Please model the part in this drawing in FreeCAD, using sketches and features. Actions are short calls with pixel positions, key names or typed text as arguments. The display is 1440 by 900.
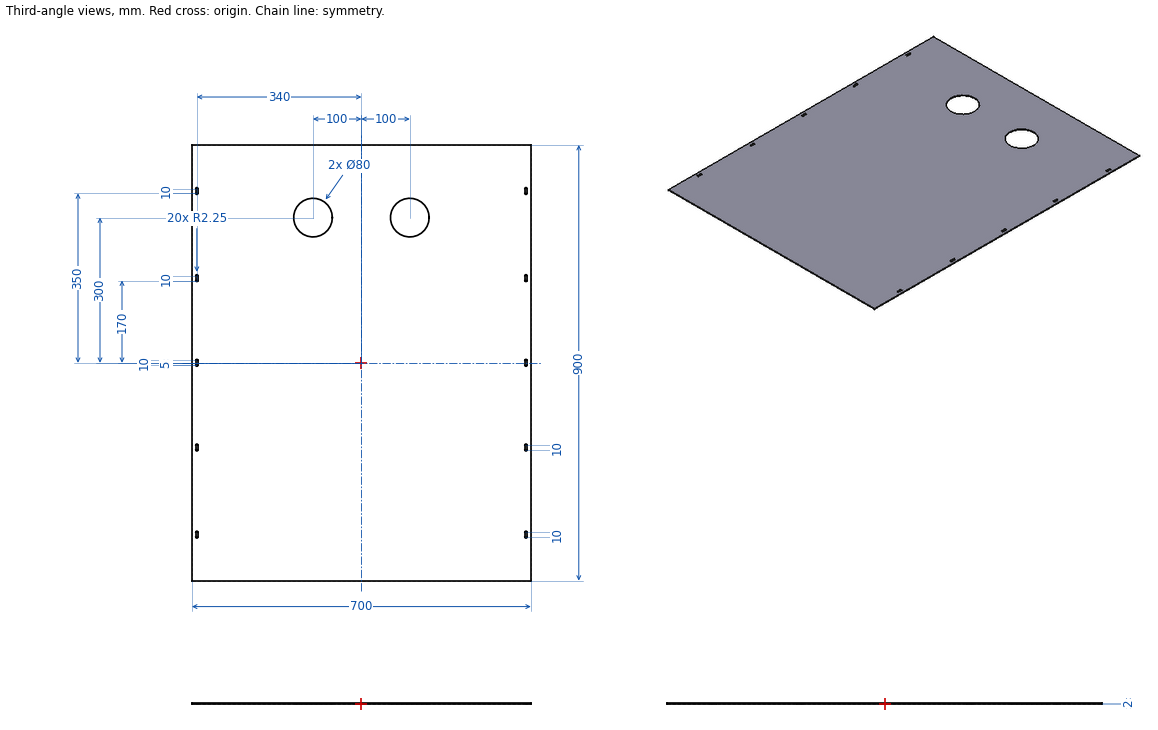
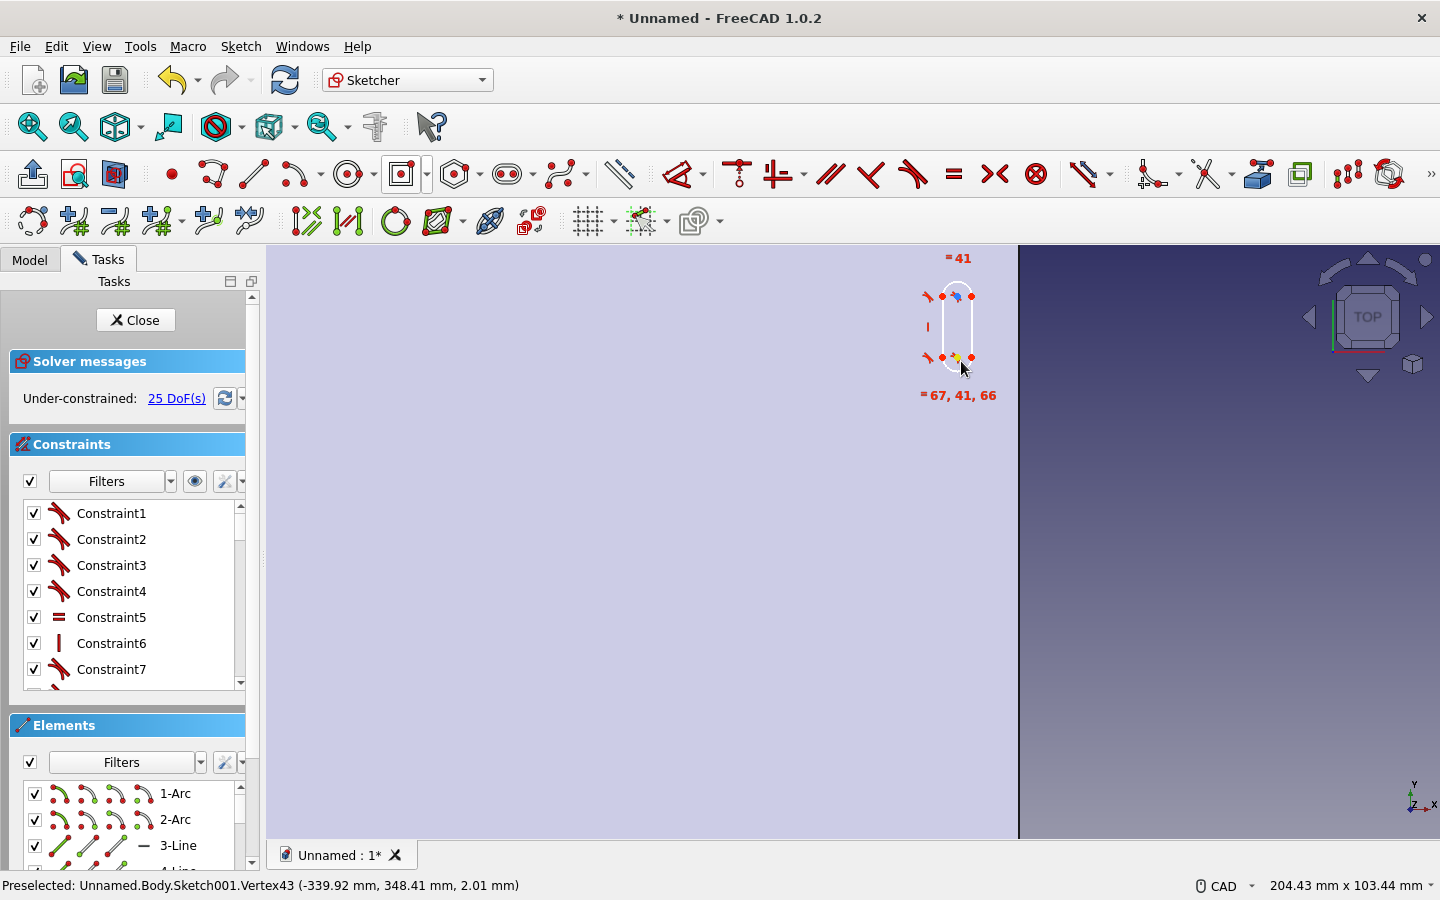
click(957, 357)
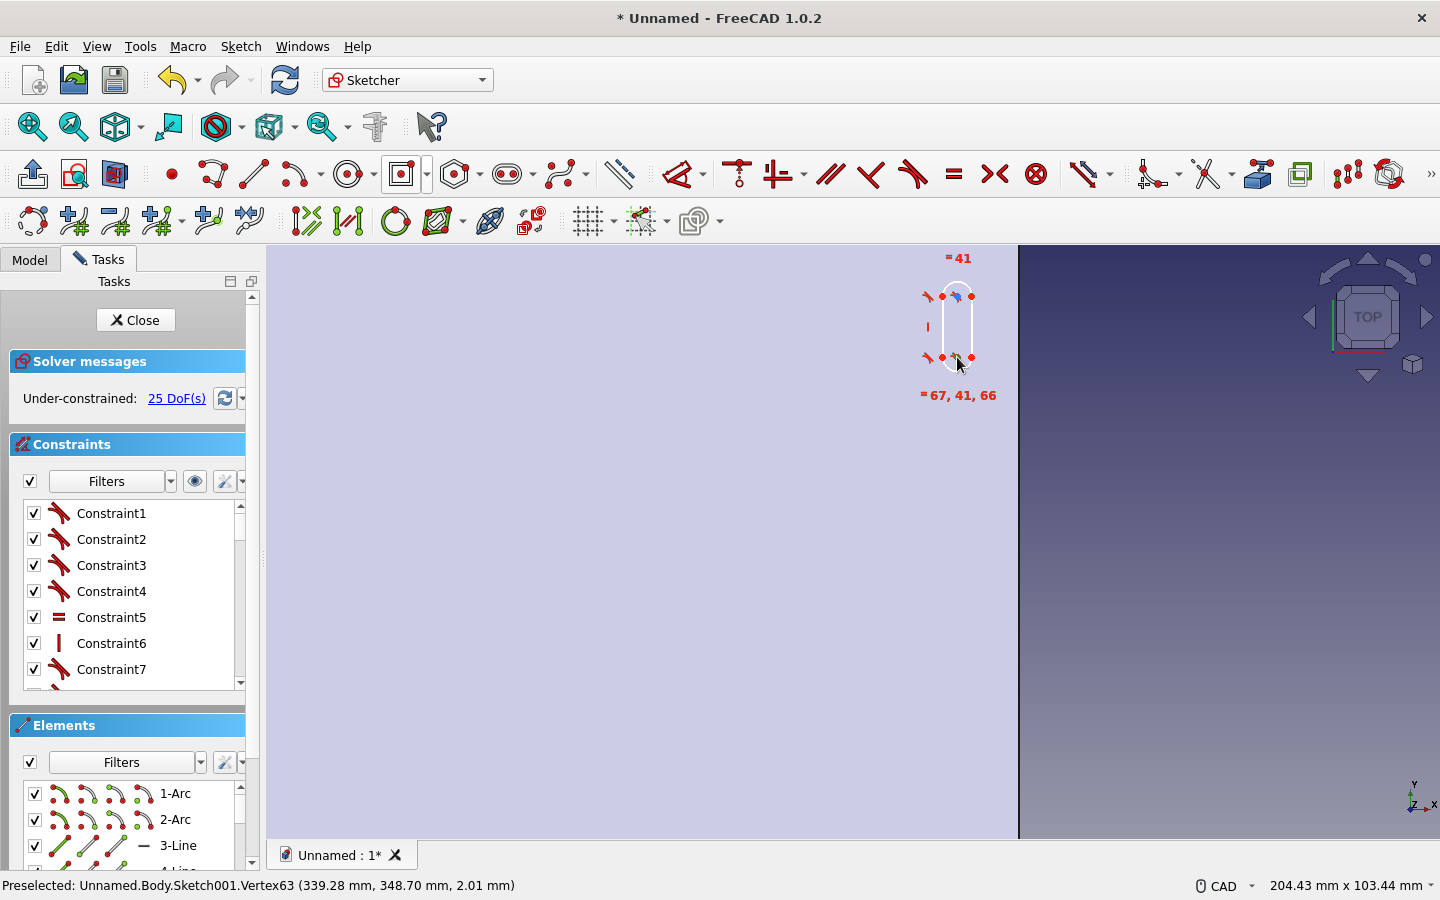
scroll(962, 361, down, 12)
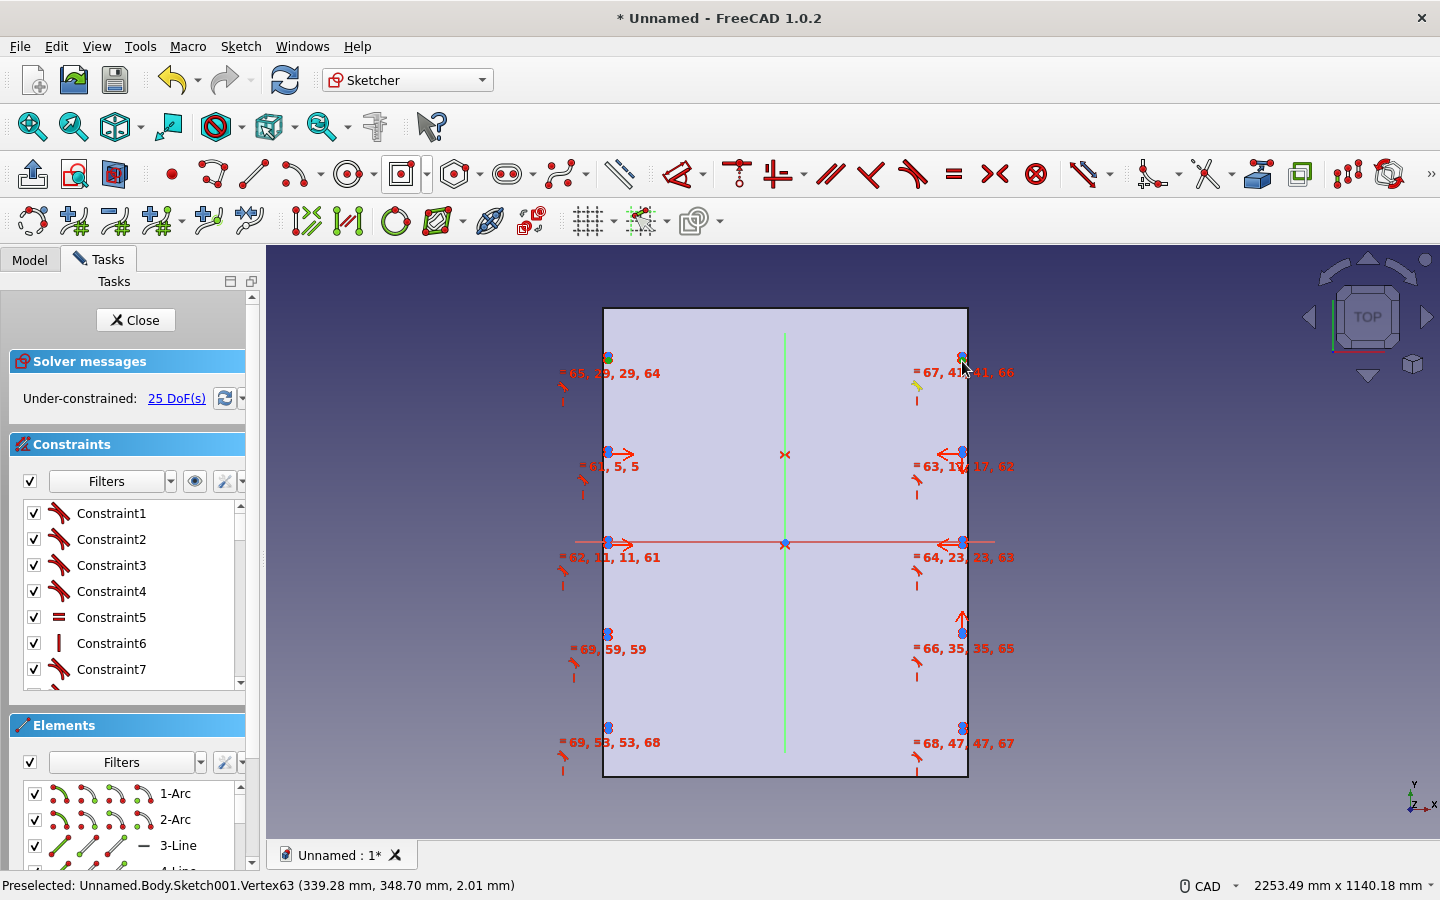
click(785, 734)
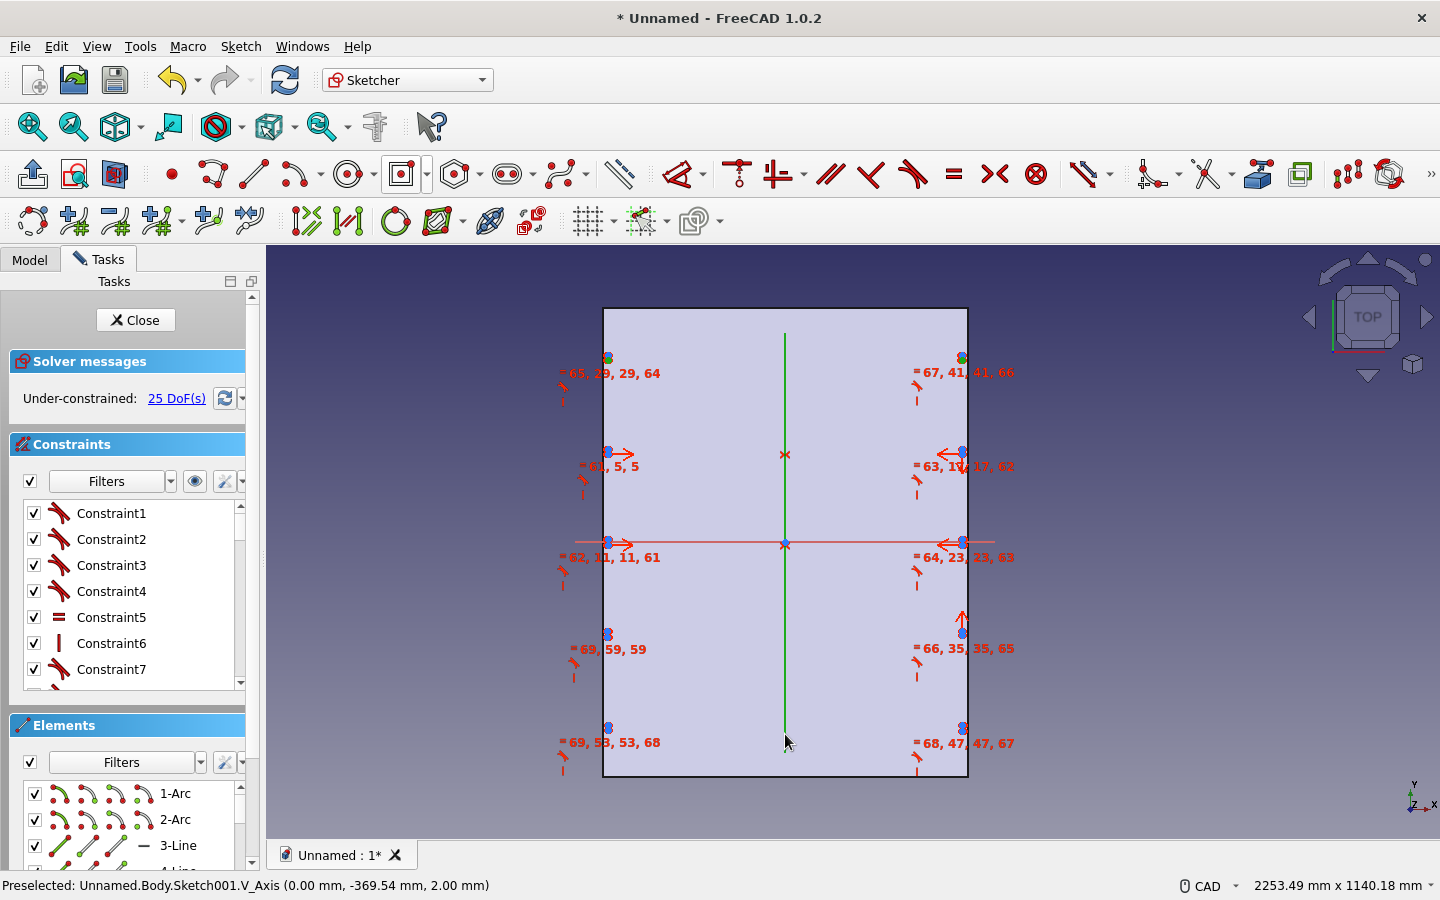
key(s)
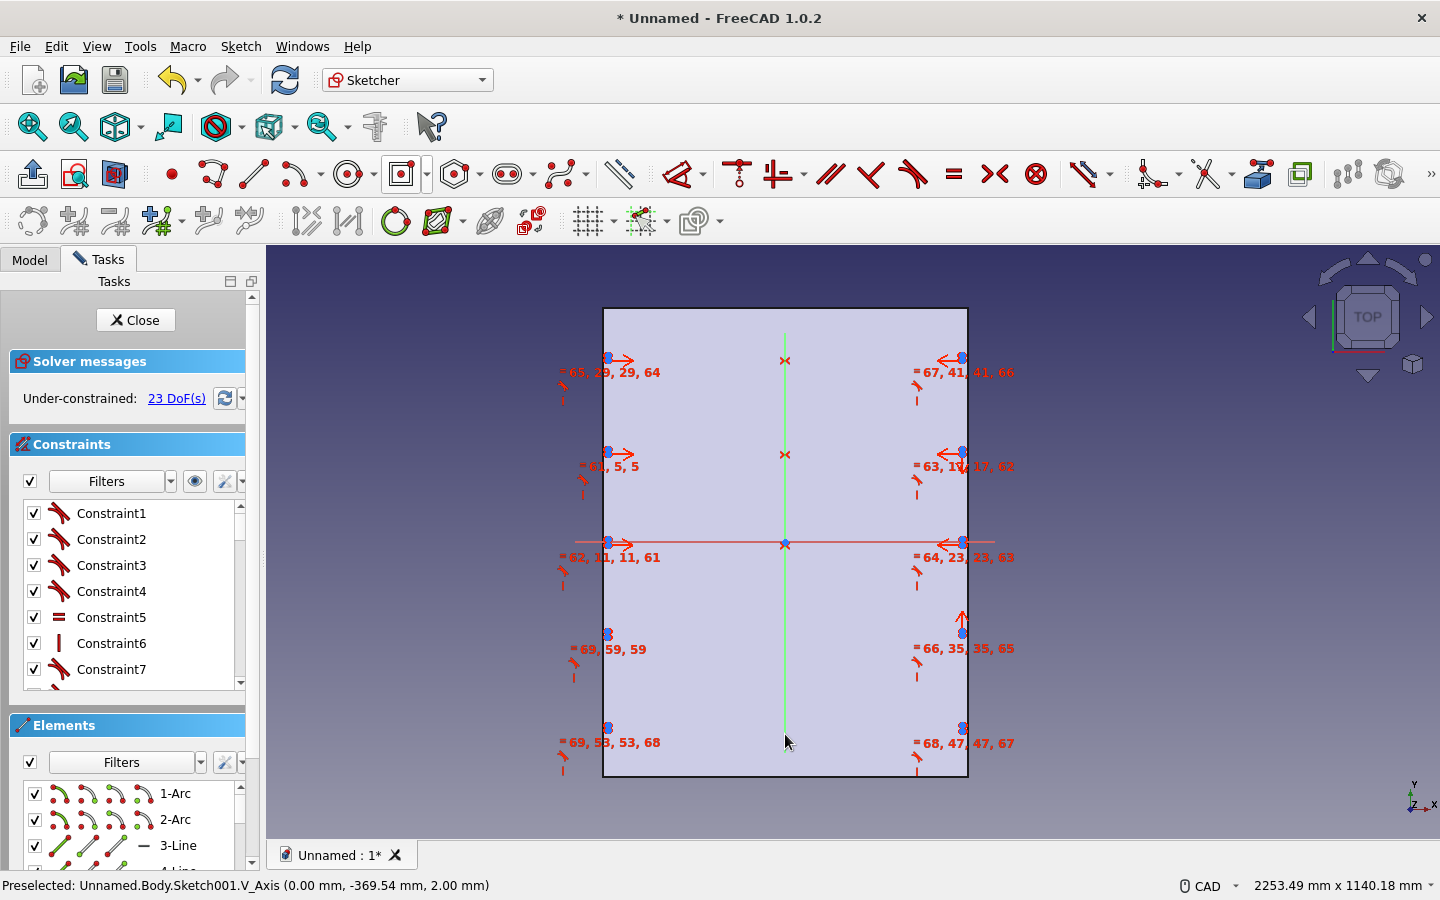
scroll(962, 355, up, 11)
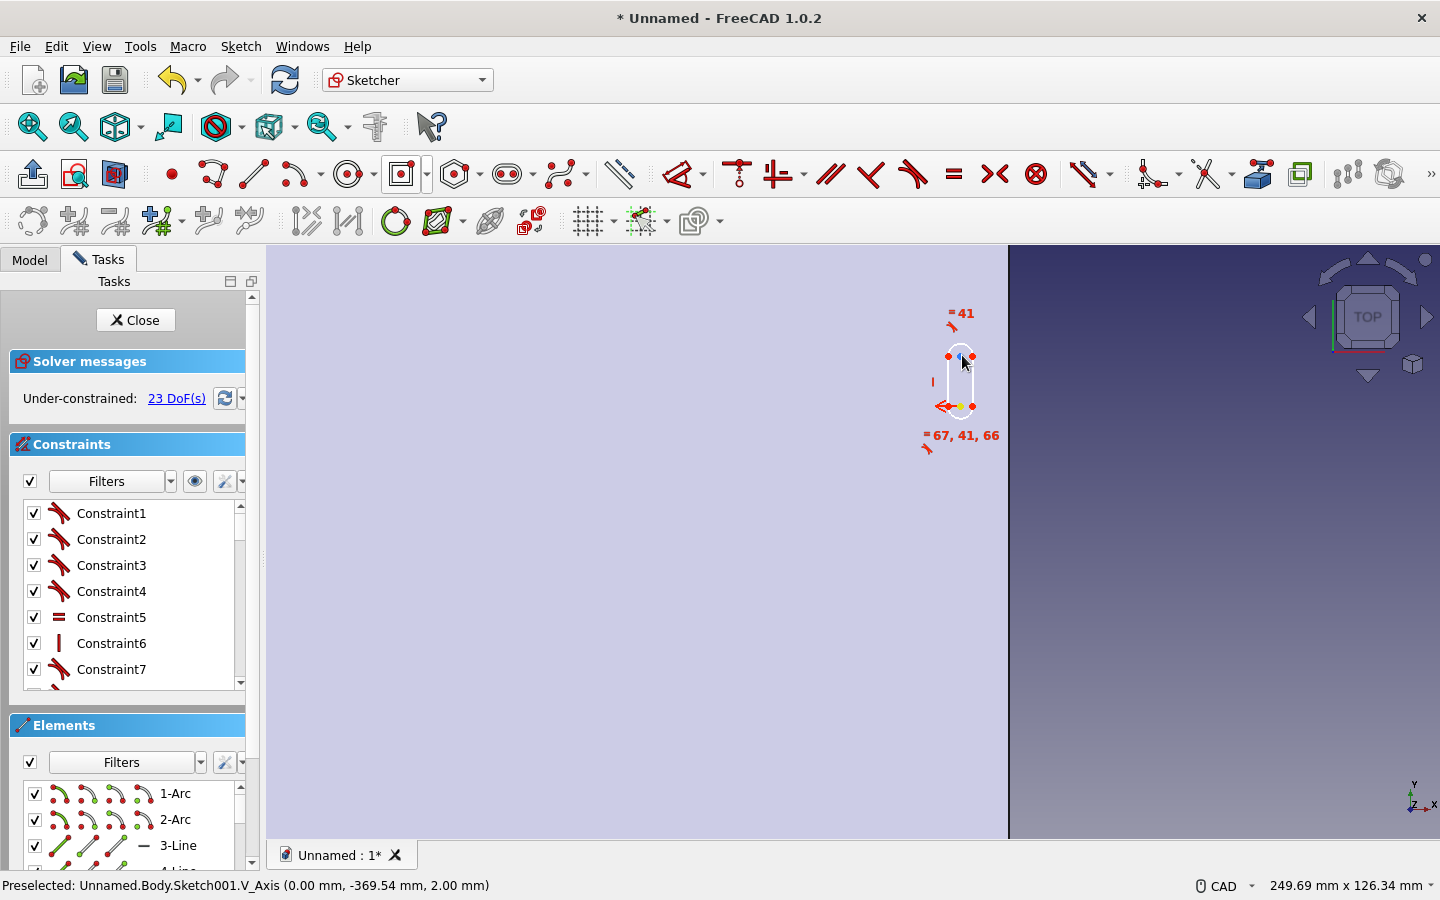
click(961, 356)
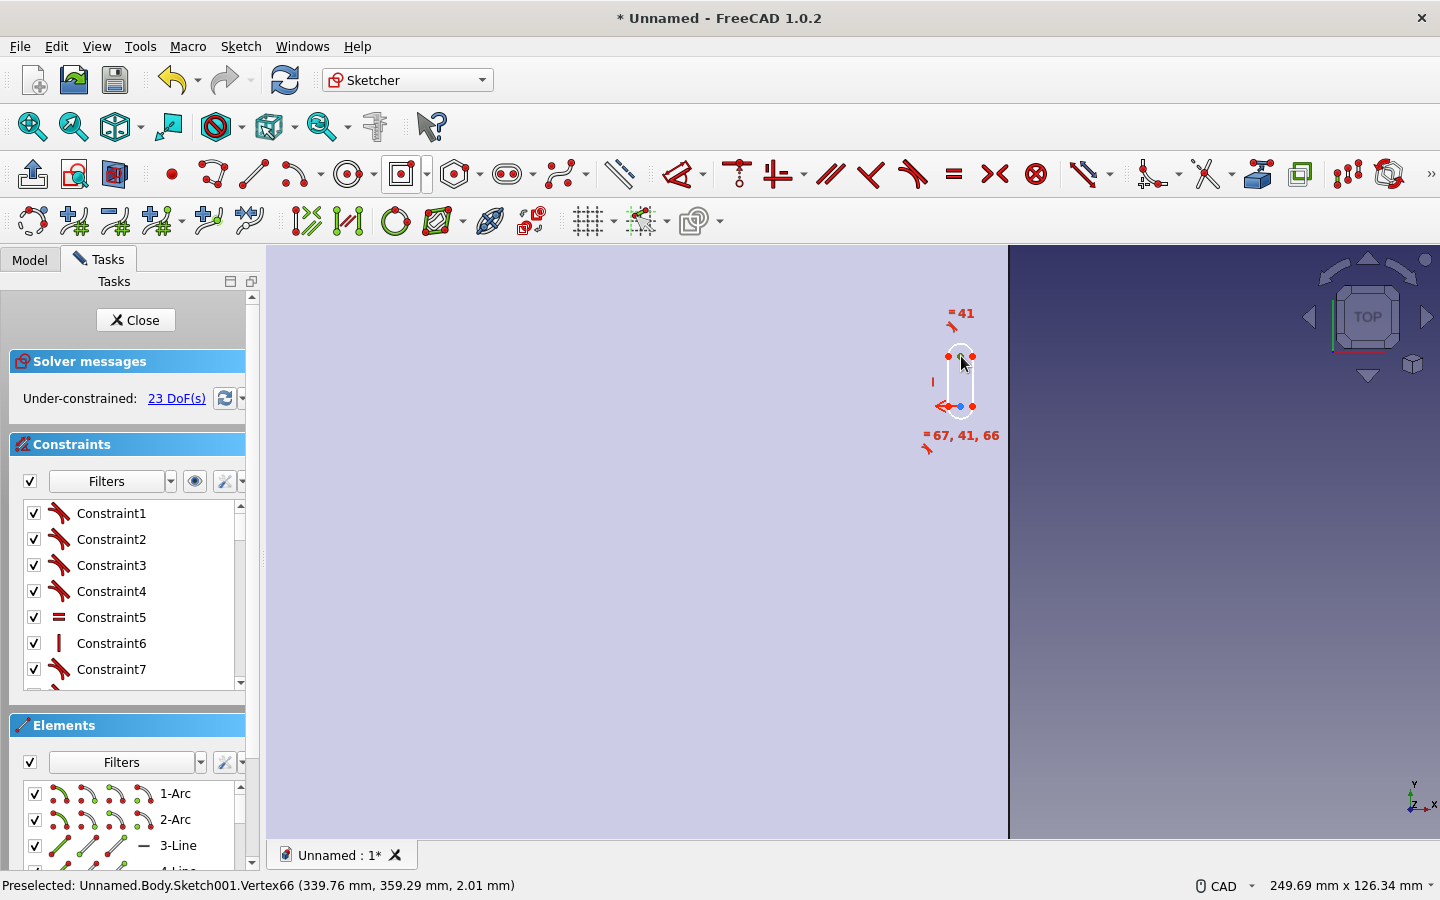
scroll(962, 355, down, 11)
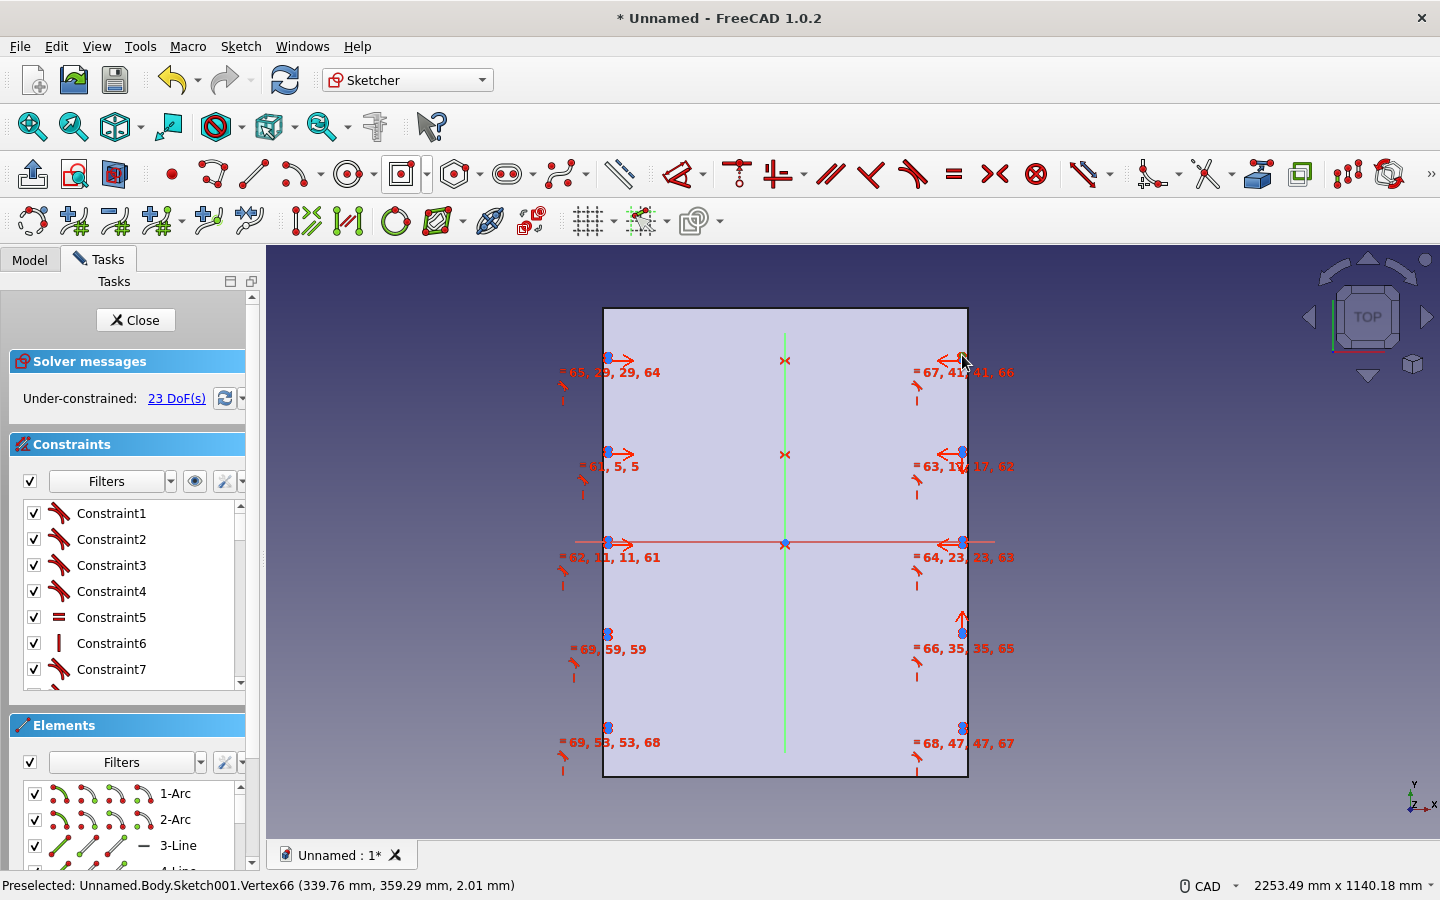
scroll(963, 731, up, 11)